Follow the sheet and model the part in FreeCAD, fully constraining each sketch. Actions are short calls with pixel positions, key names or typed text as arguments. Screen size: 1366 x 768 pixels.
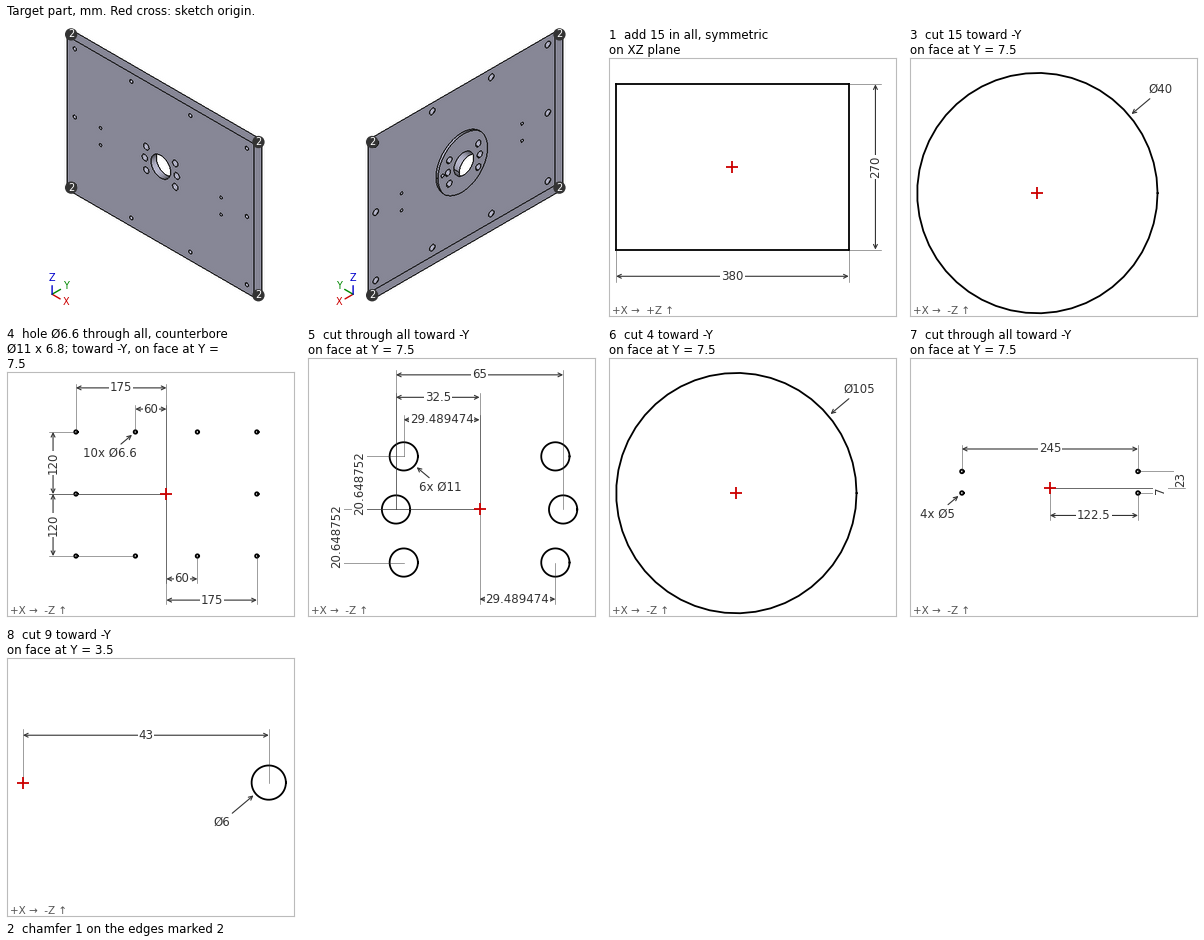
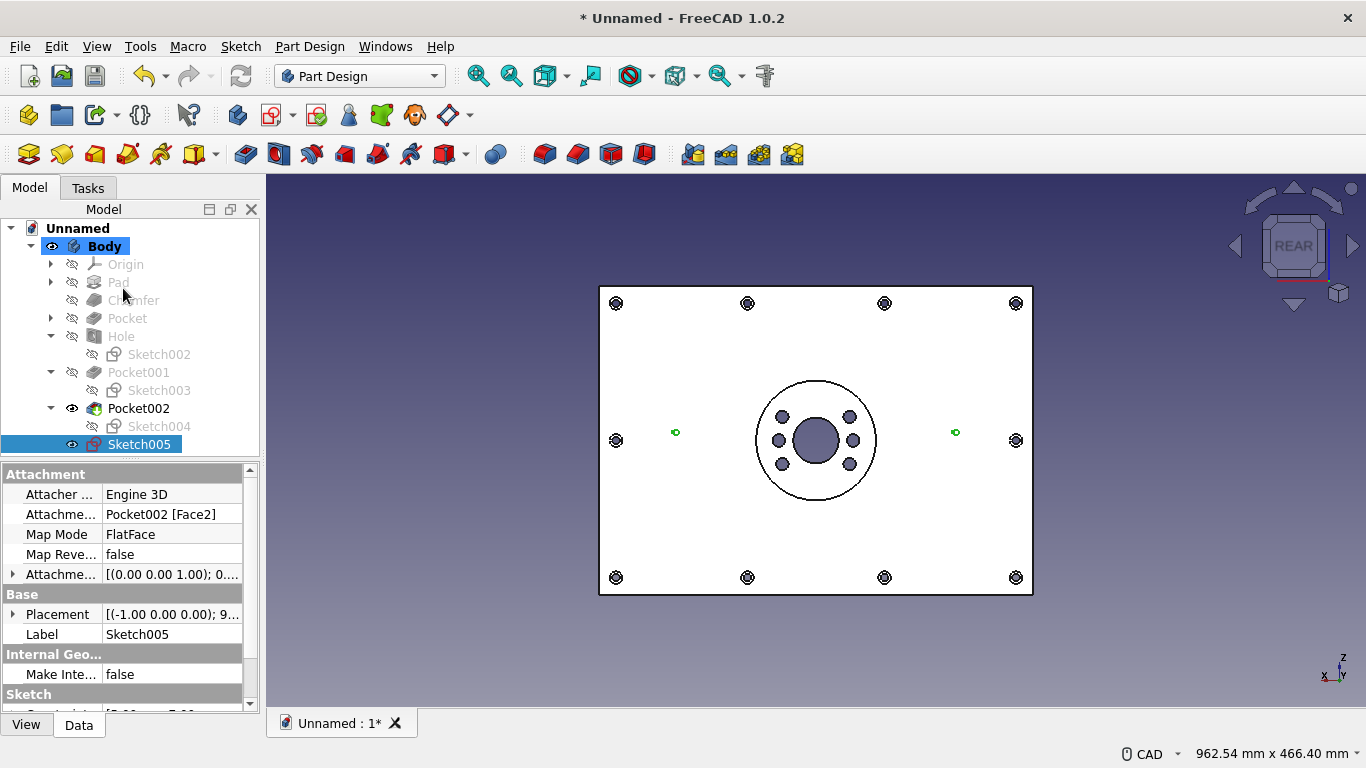
click(246, 154)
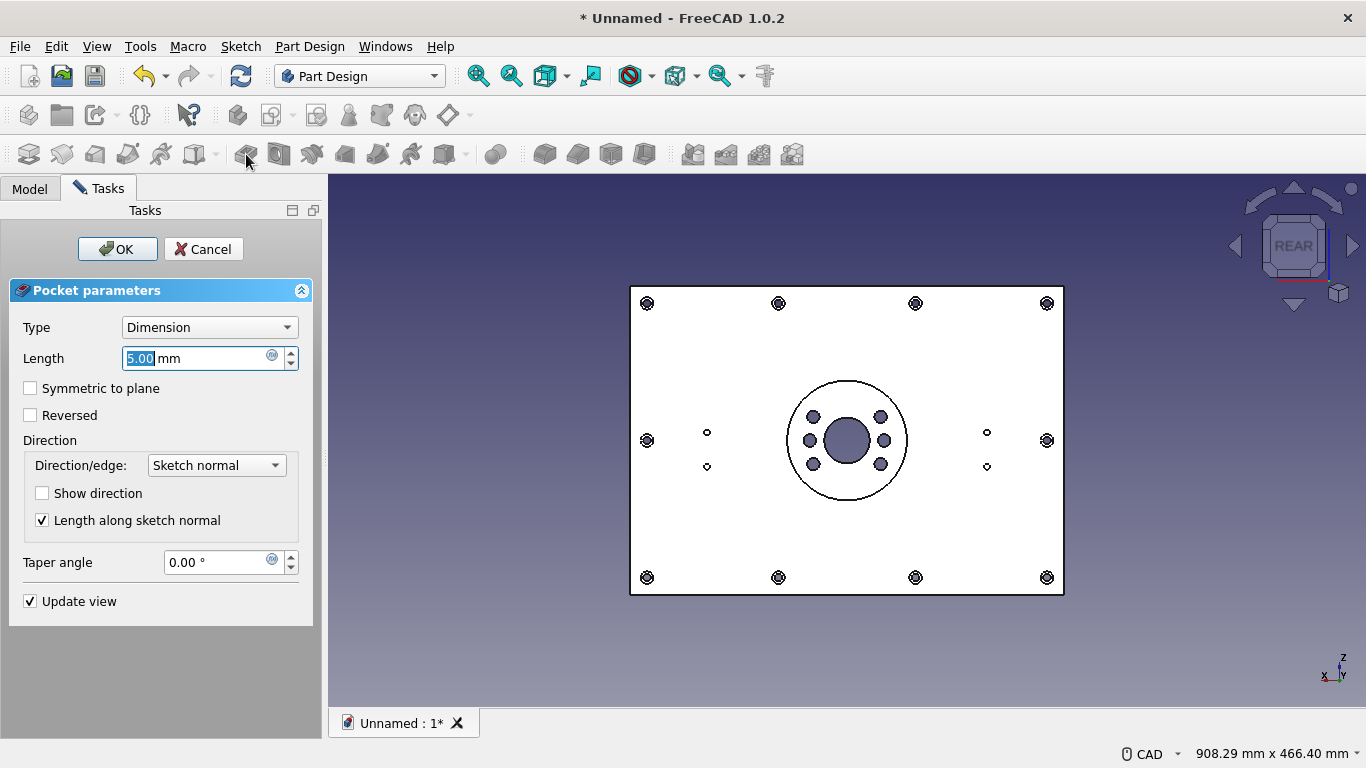
click(210, 328)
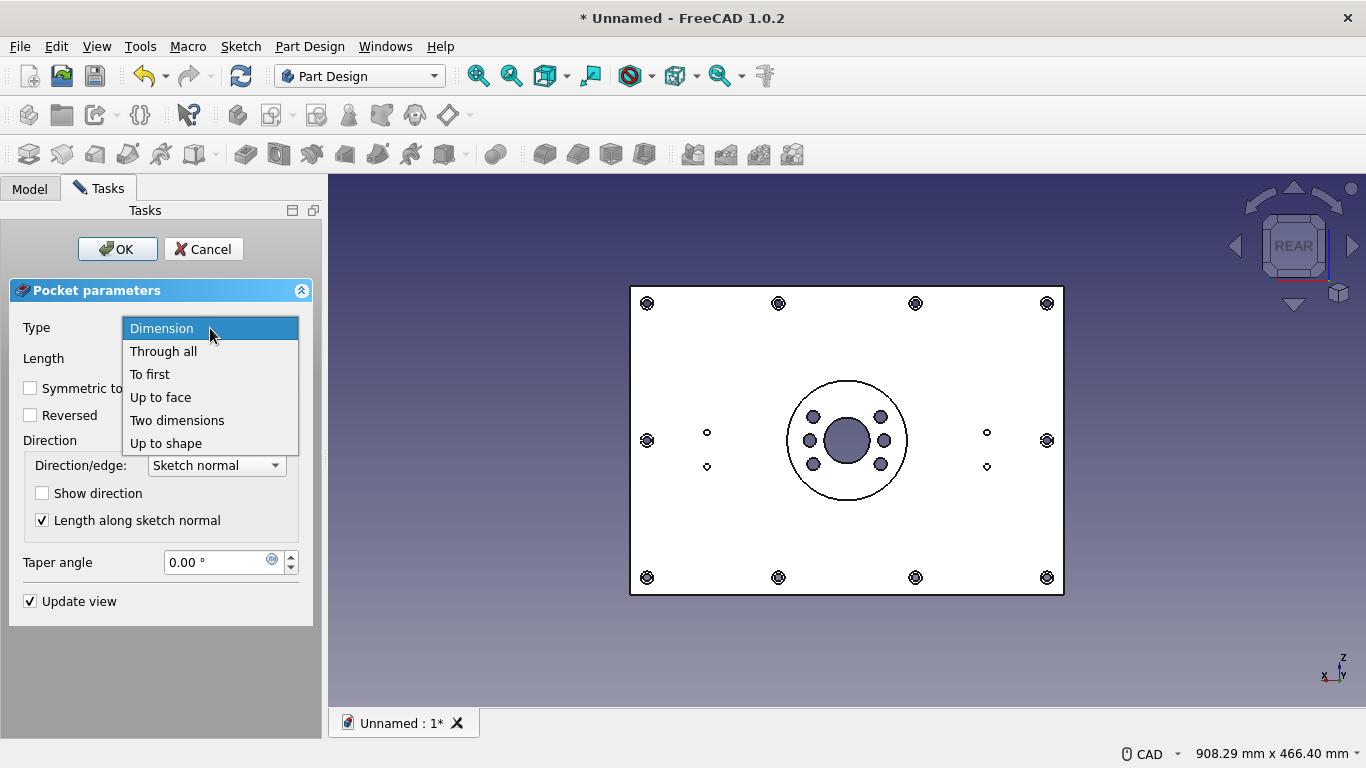
click(208, 352)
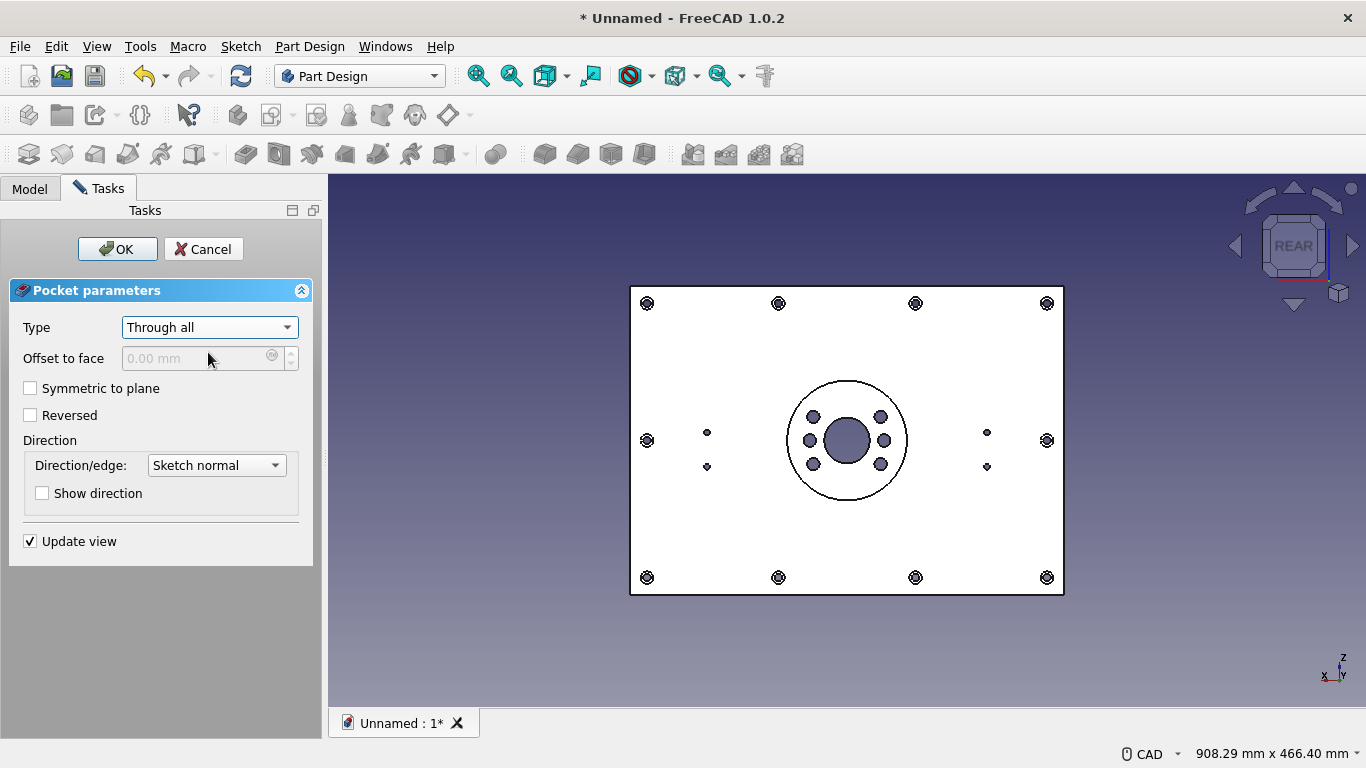
click(118, 249)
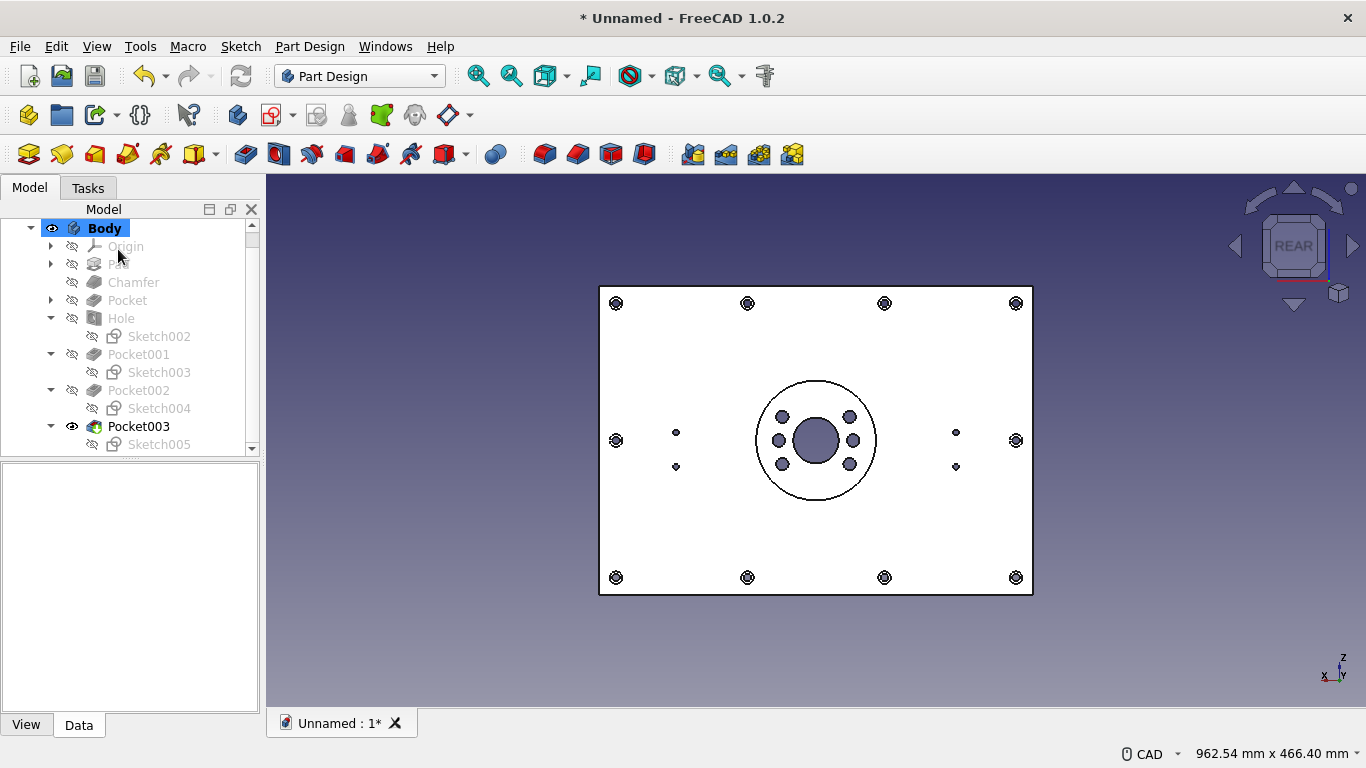
click(799, 474)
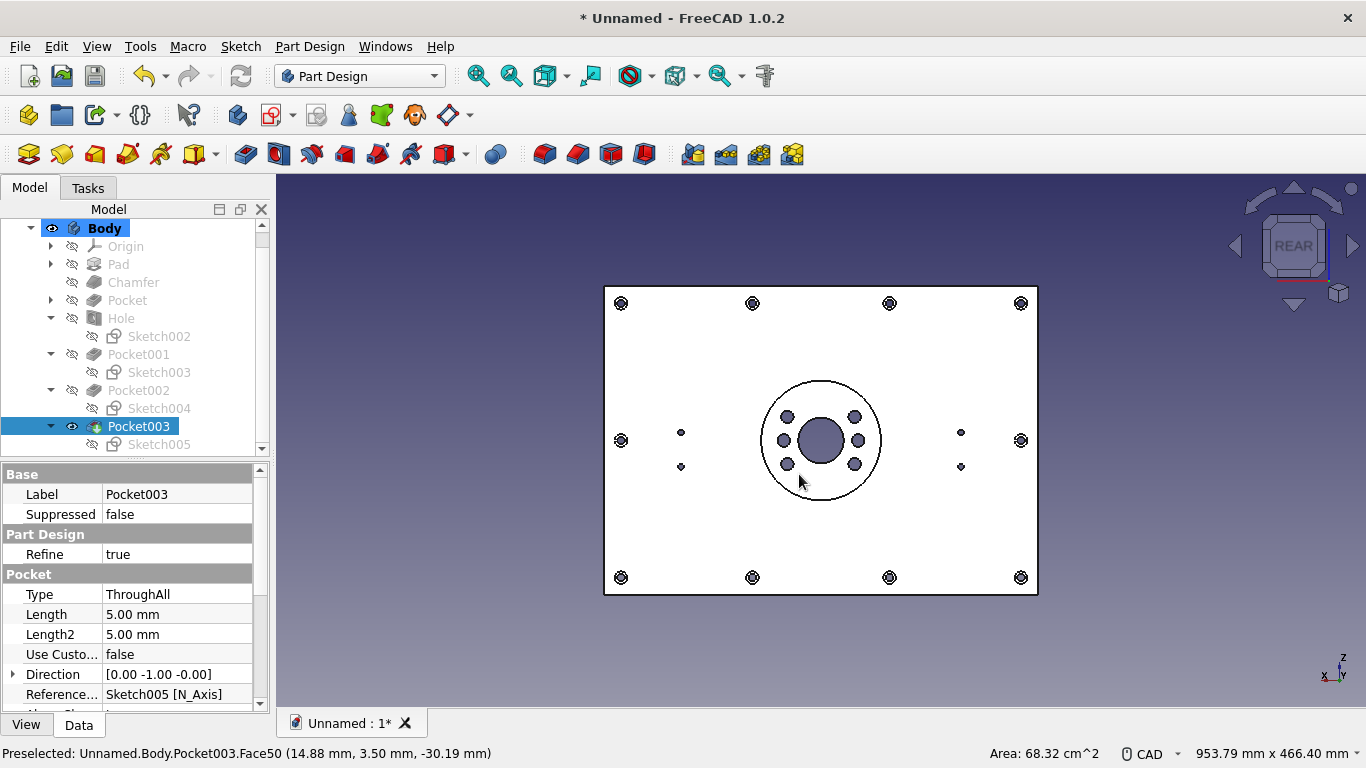
click(270, 116)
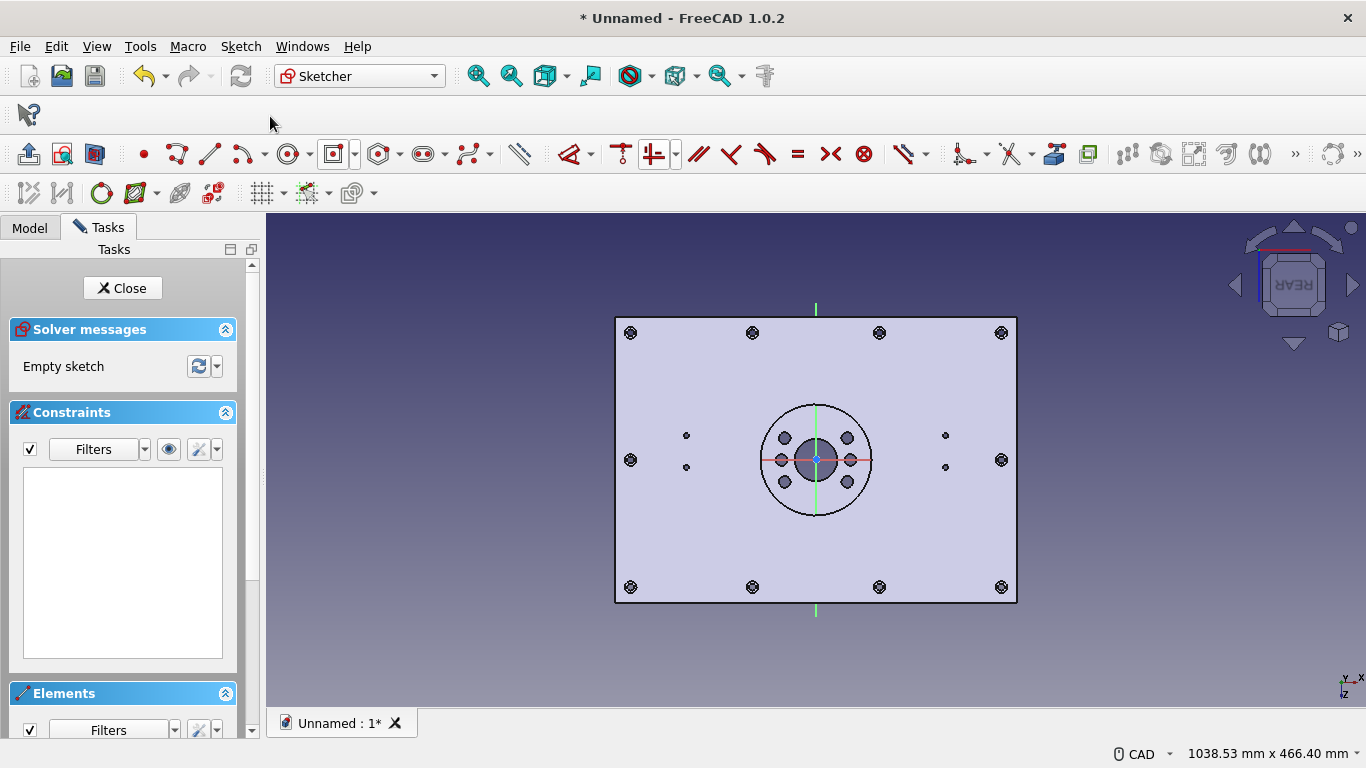
click(95, 154)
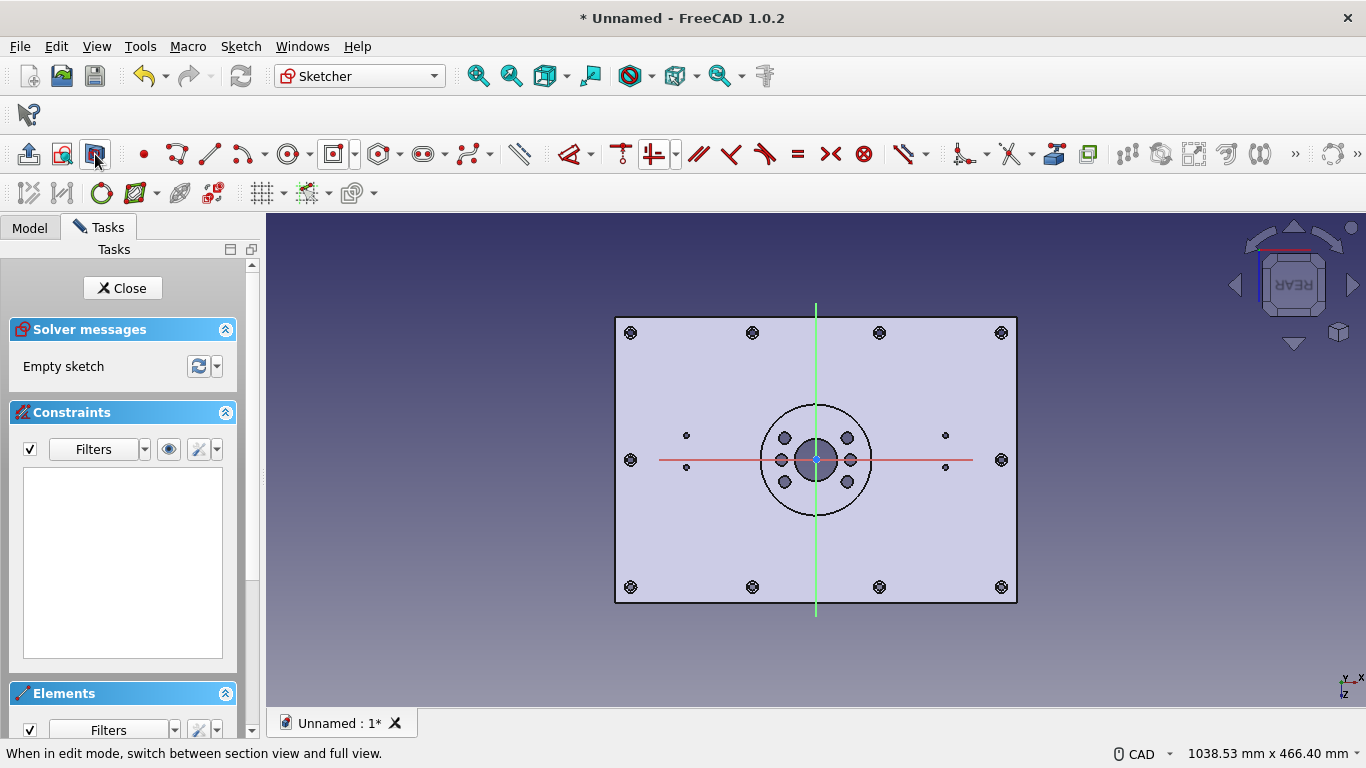
scroll(868, 460, up, 15)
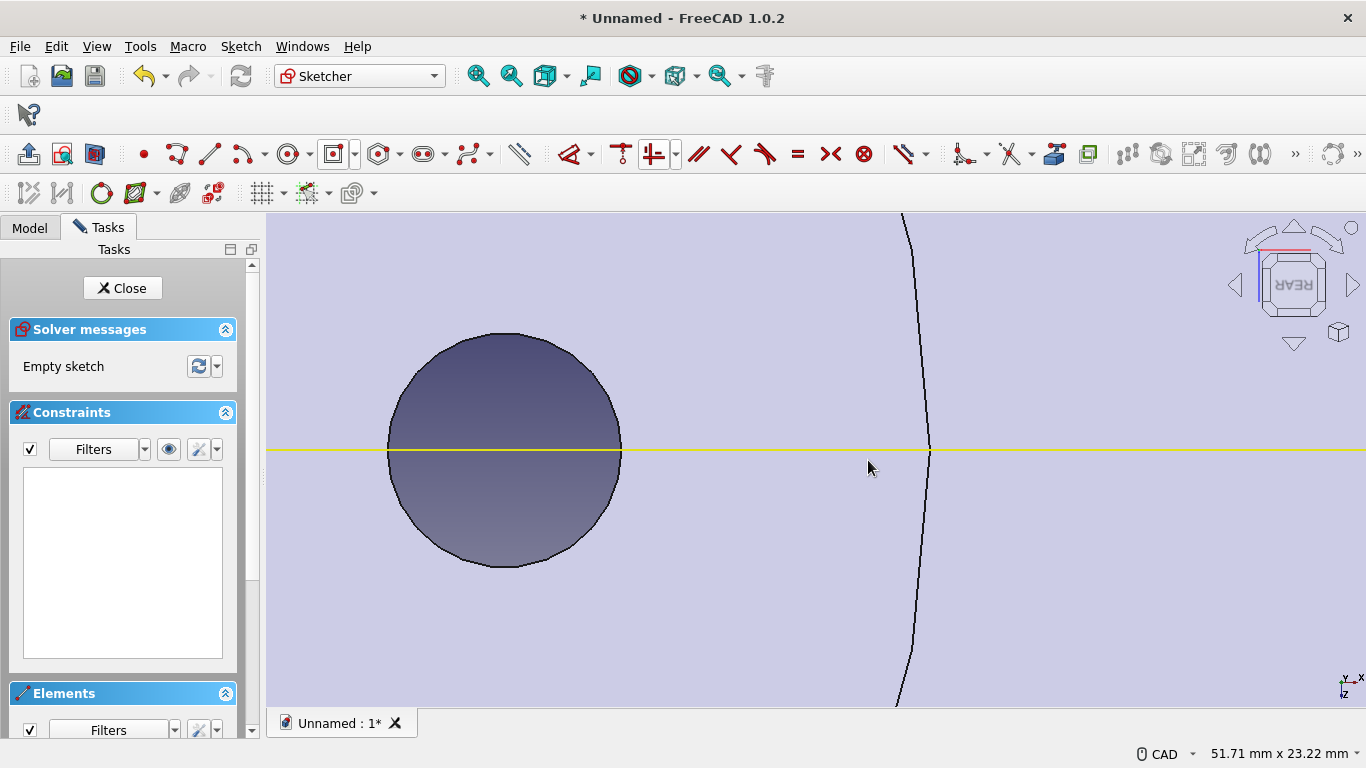
scroll(712, 443, up, 4)